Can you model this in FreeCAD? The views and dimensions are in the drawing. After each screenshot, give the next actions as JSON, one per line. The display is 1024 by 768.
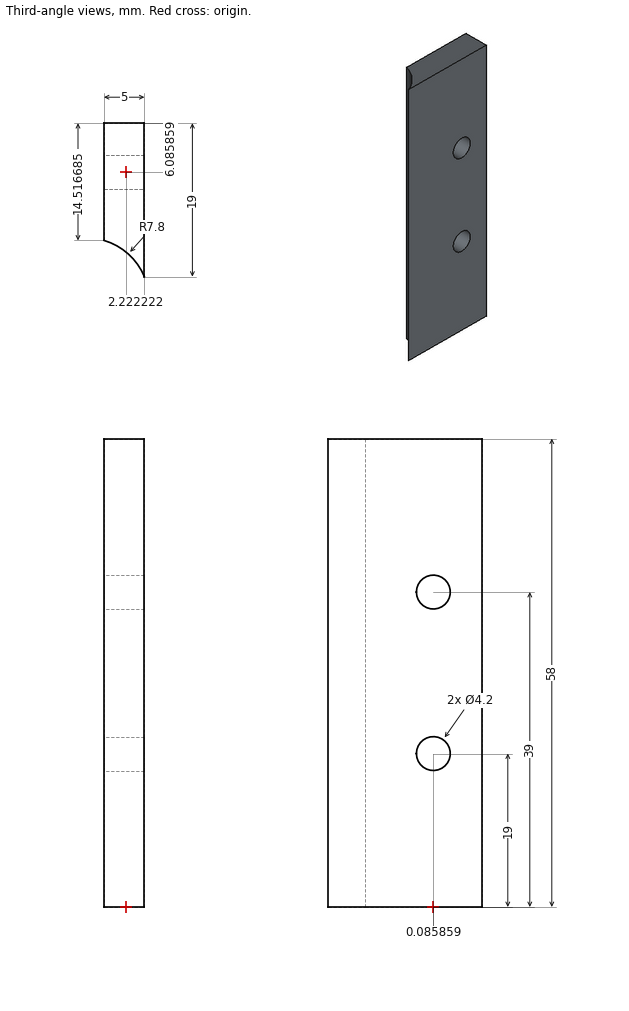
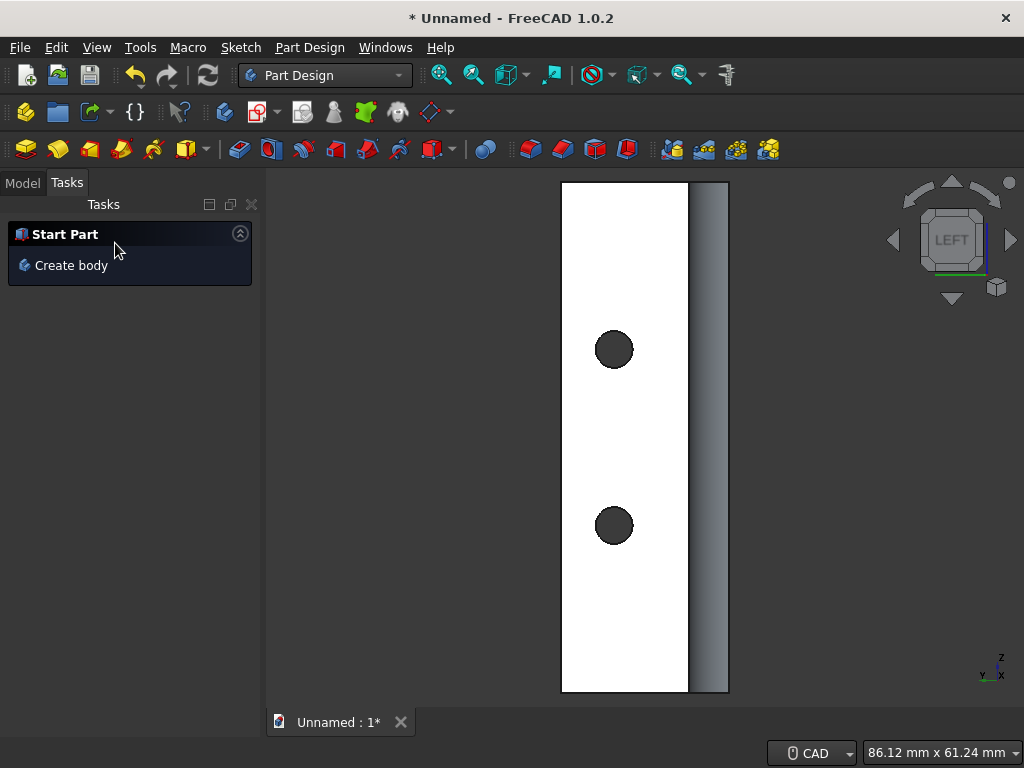
{"action": "key", "text": "0"}